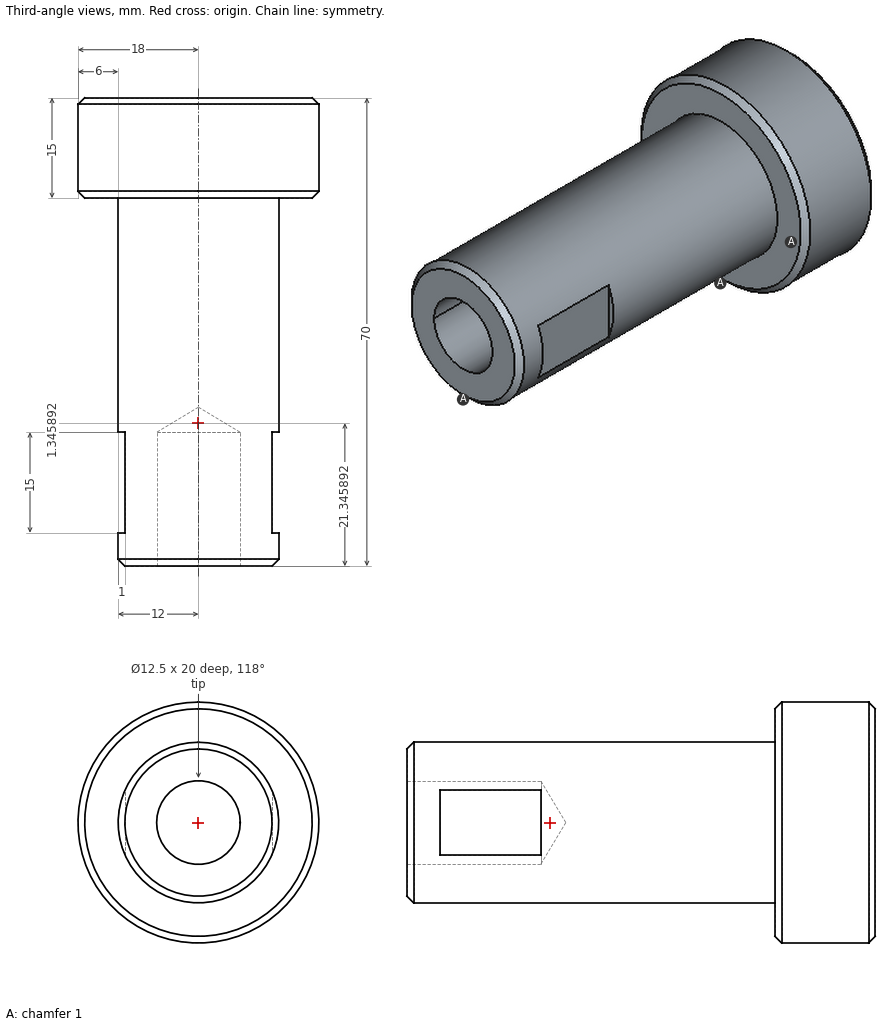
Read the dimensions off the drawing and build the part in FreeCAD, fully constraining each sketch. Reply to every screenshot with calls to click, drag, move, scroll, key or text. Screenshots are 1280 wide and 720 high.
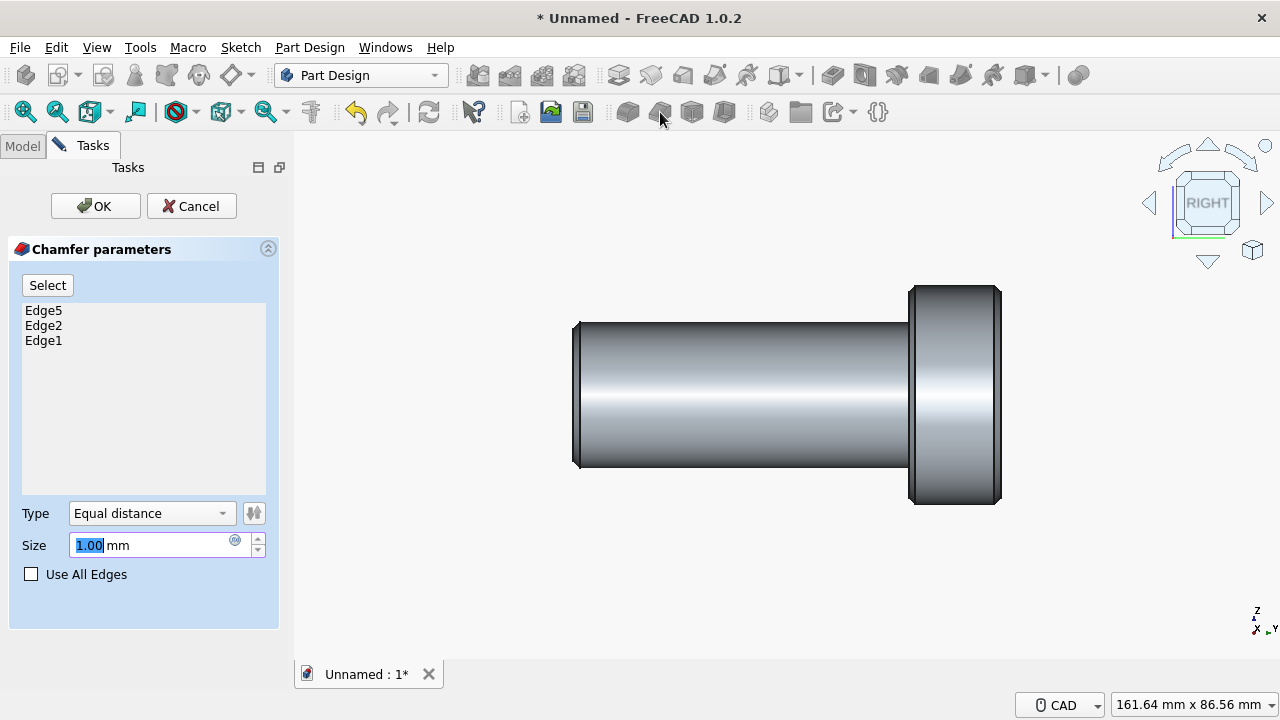
text(1)
key(Tab)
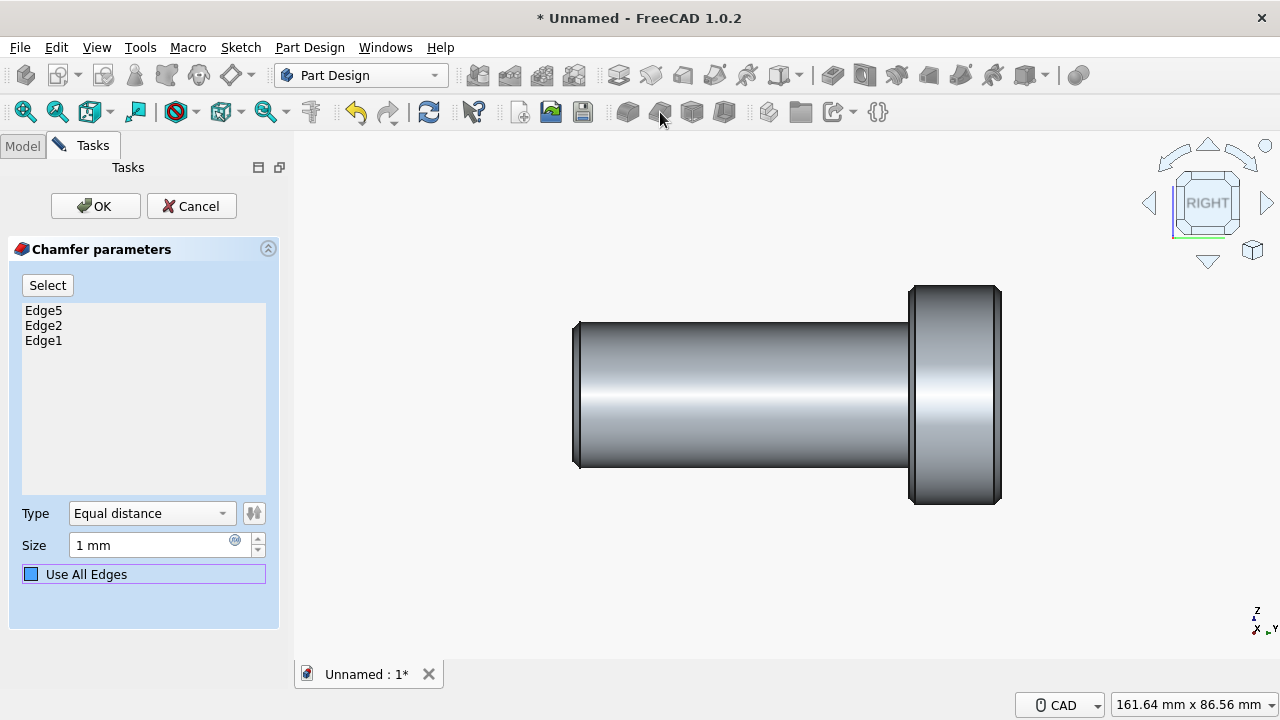
click(96, 206)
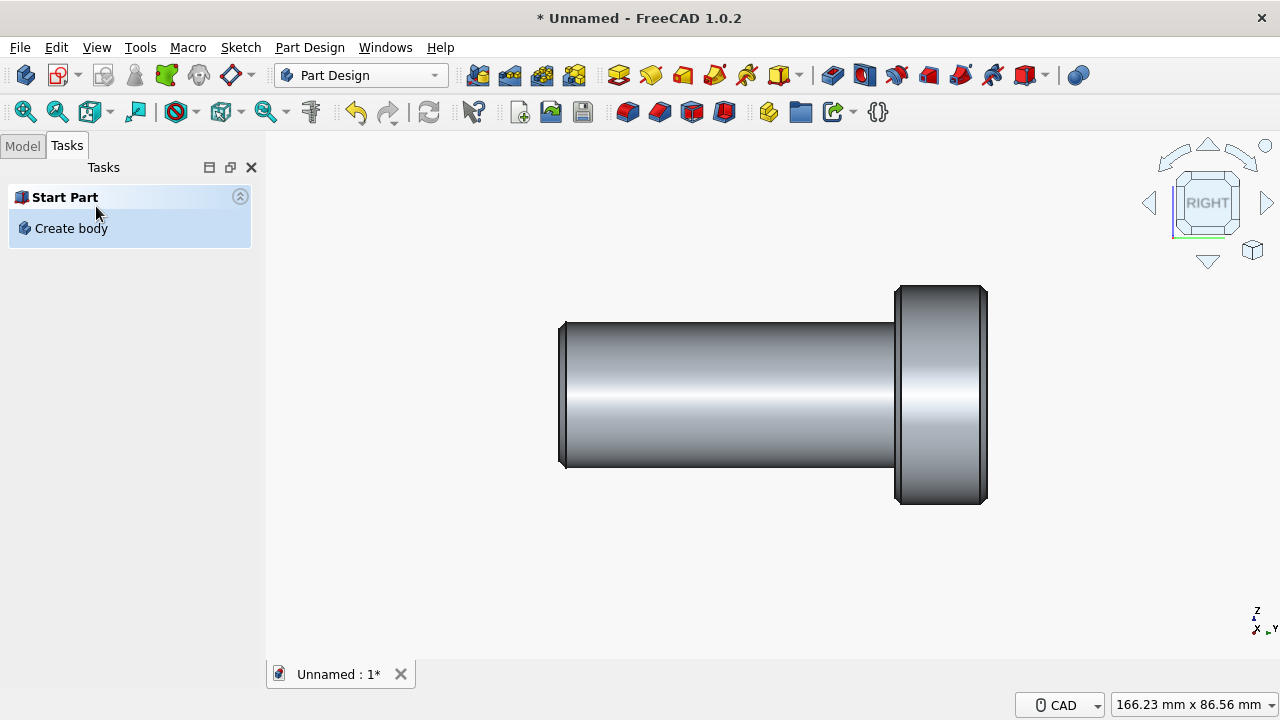
click(26, 112)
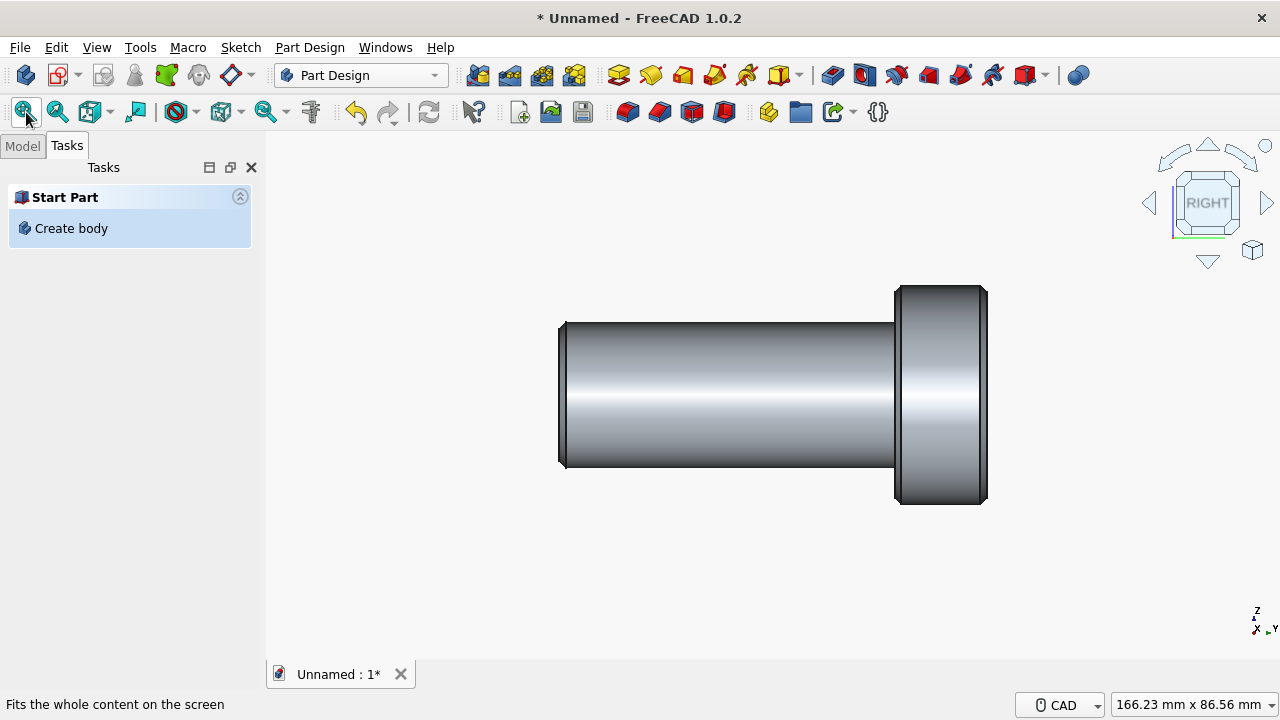
click(58, 76)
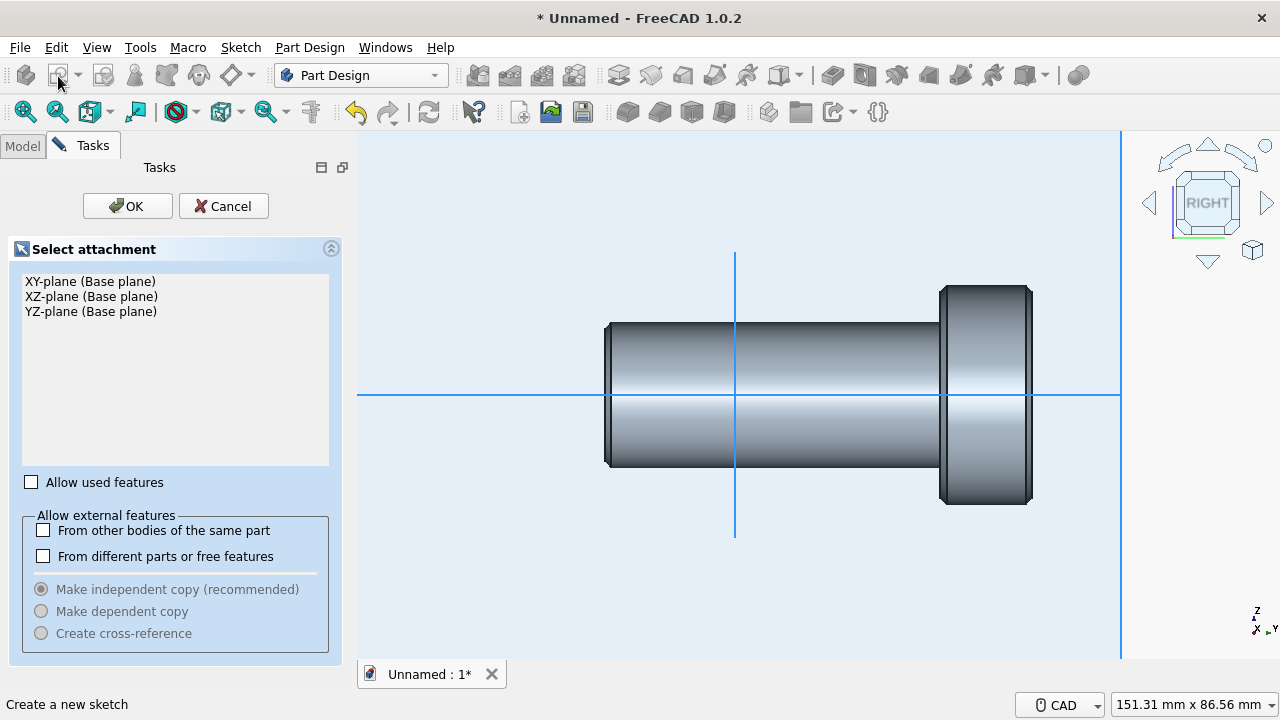
click(82, 282)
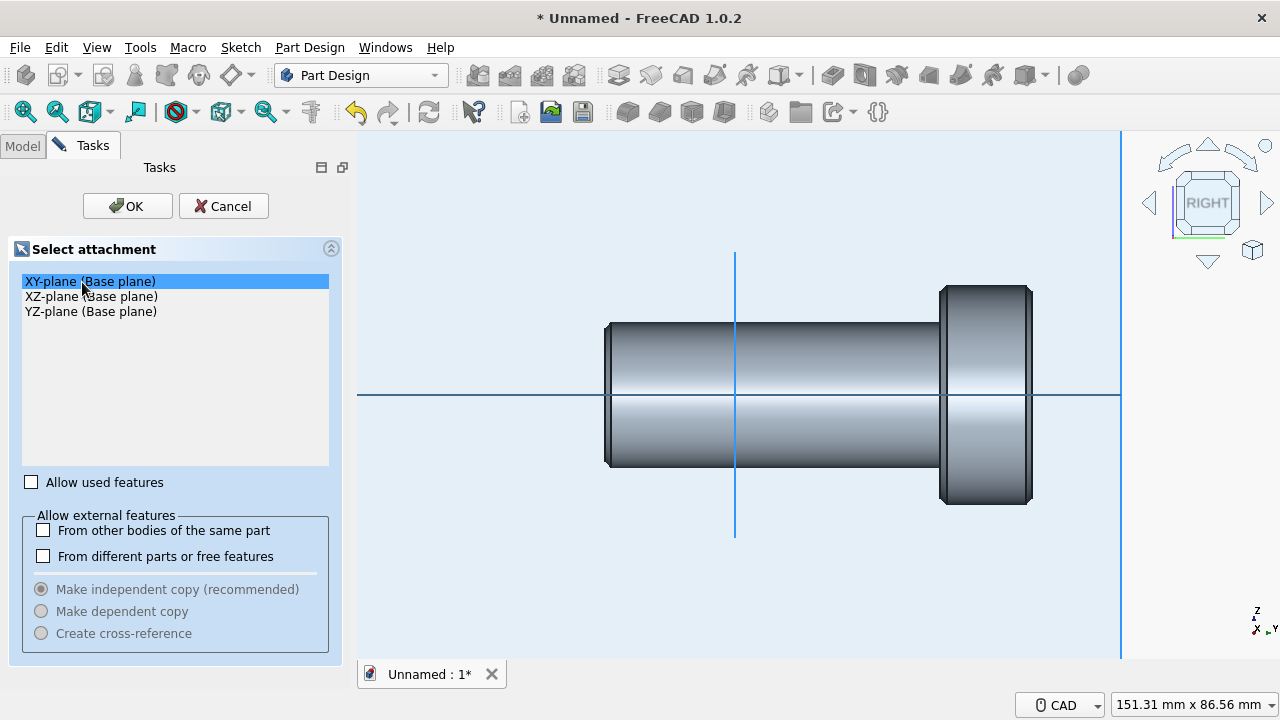
click(128, 206)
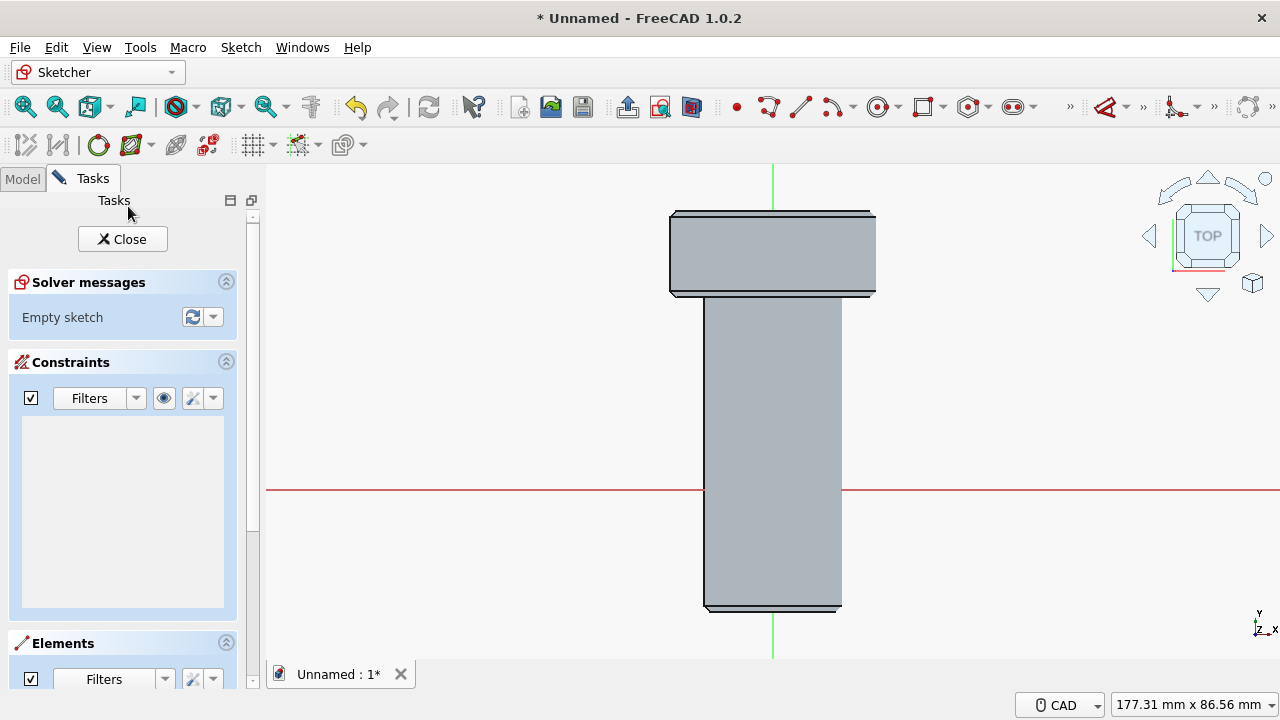
click(692, 108)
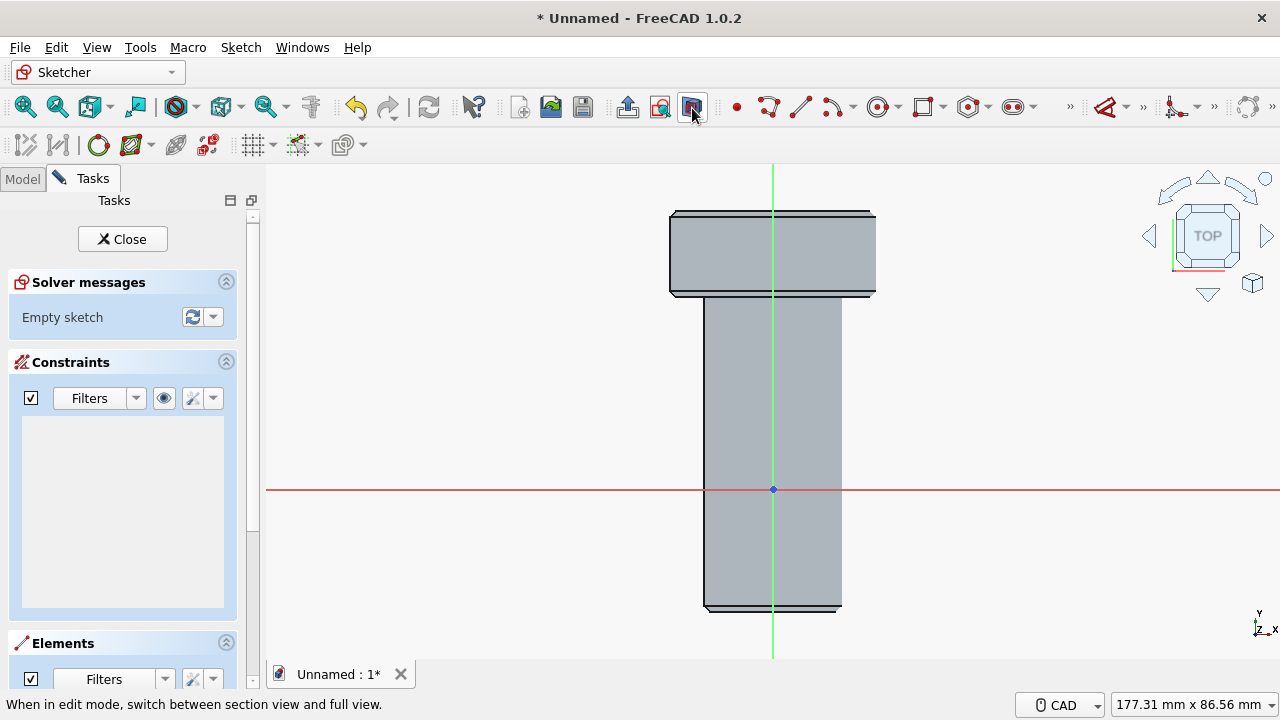
scroll(803, 590, up, 6)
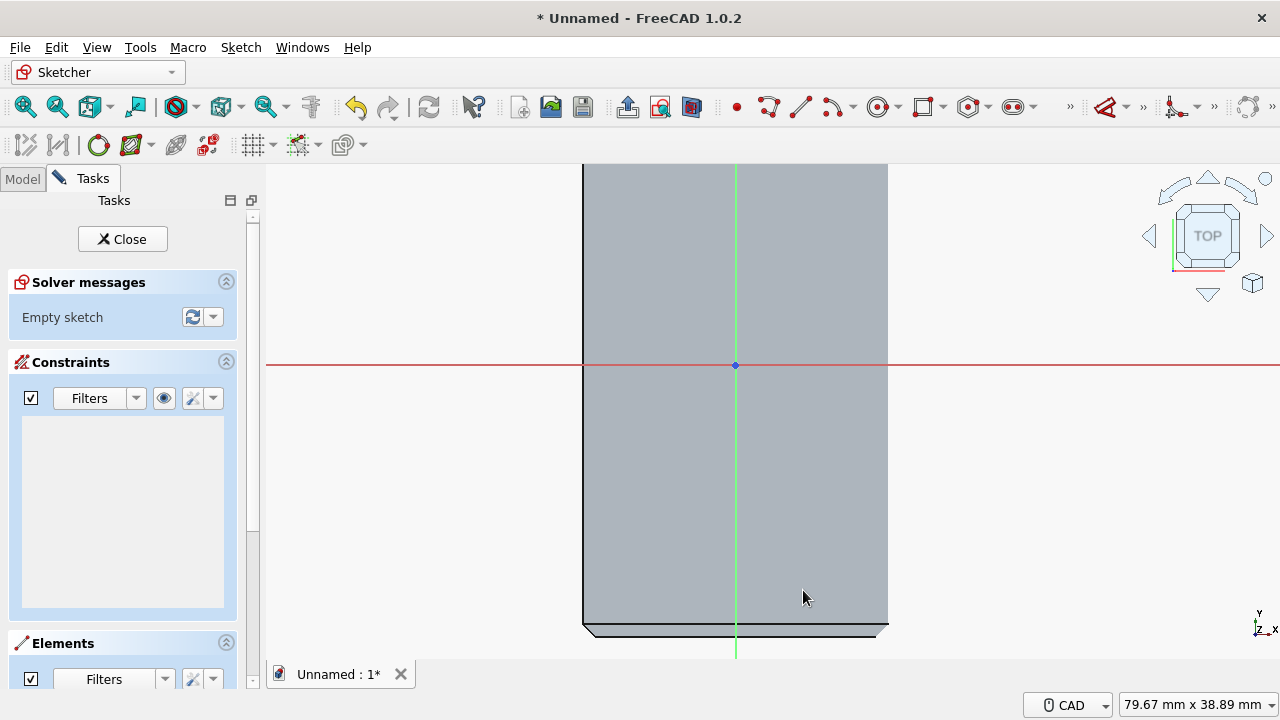
click(924, 108)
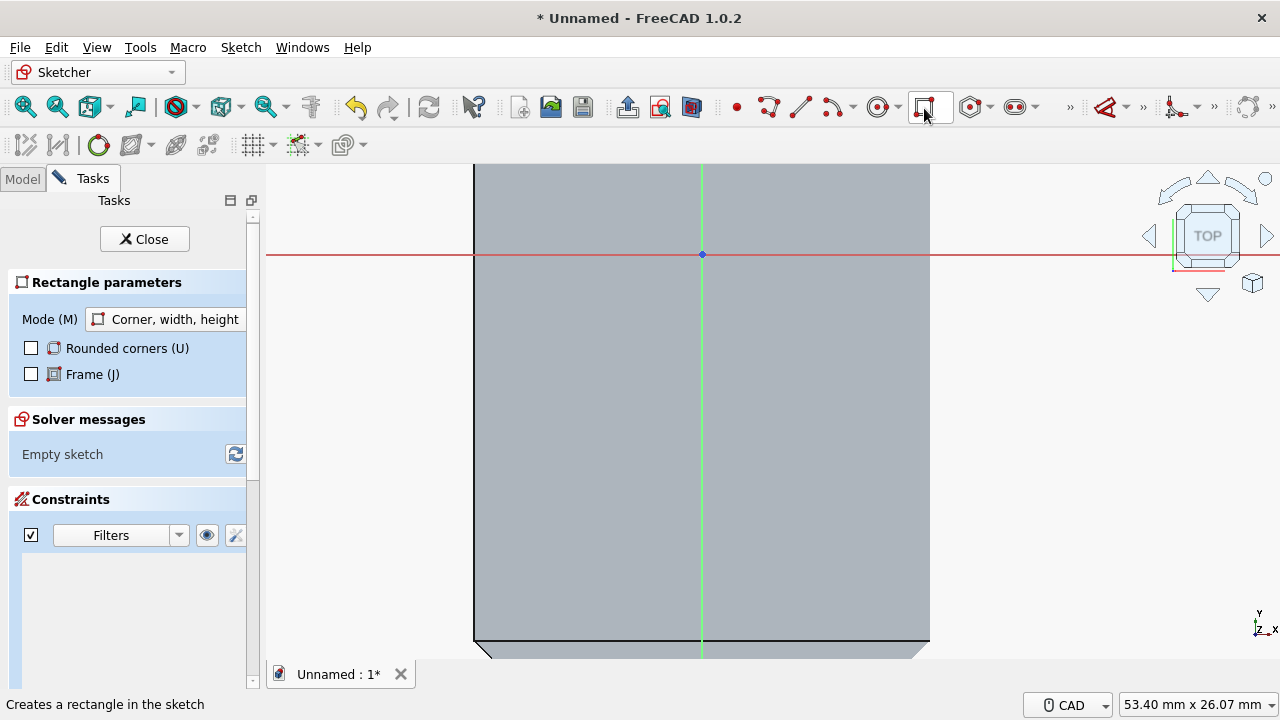
click(474, 280)
click(493, 565)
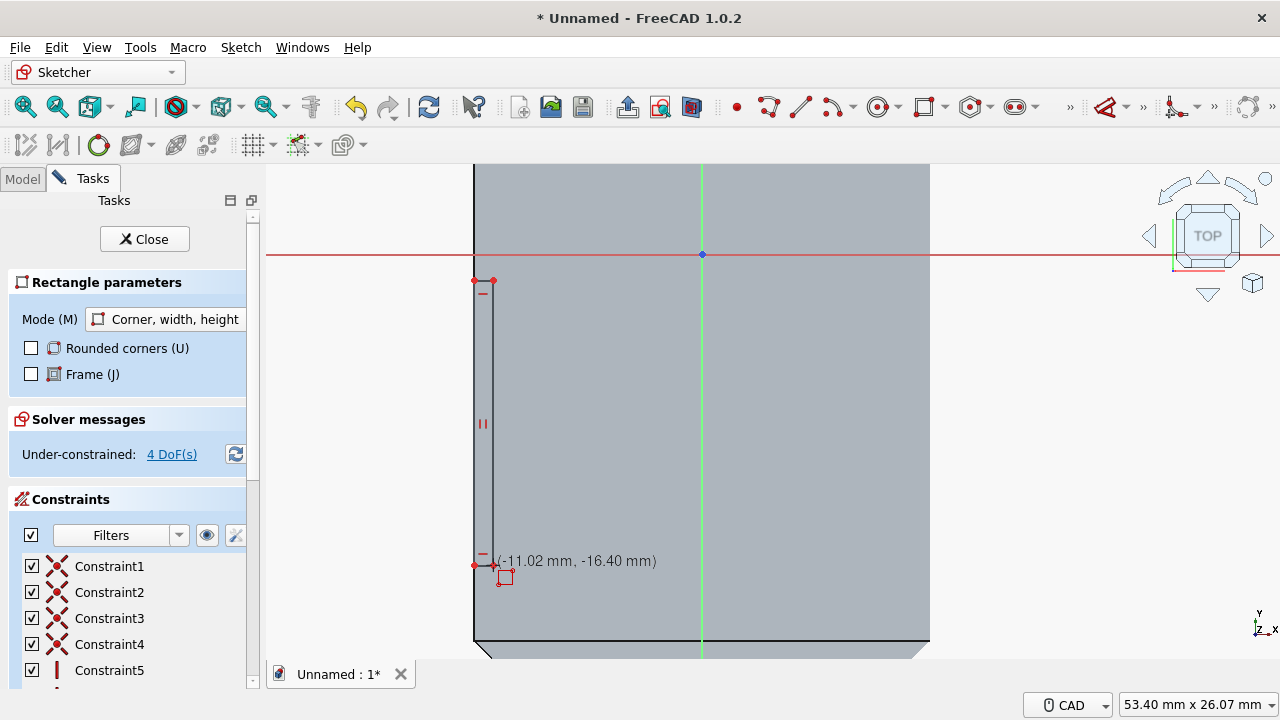
click(911, 280)
click(930, 565)
key(Escape)